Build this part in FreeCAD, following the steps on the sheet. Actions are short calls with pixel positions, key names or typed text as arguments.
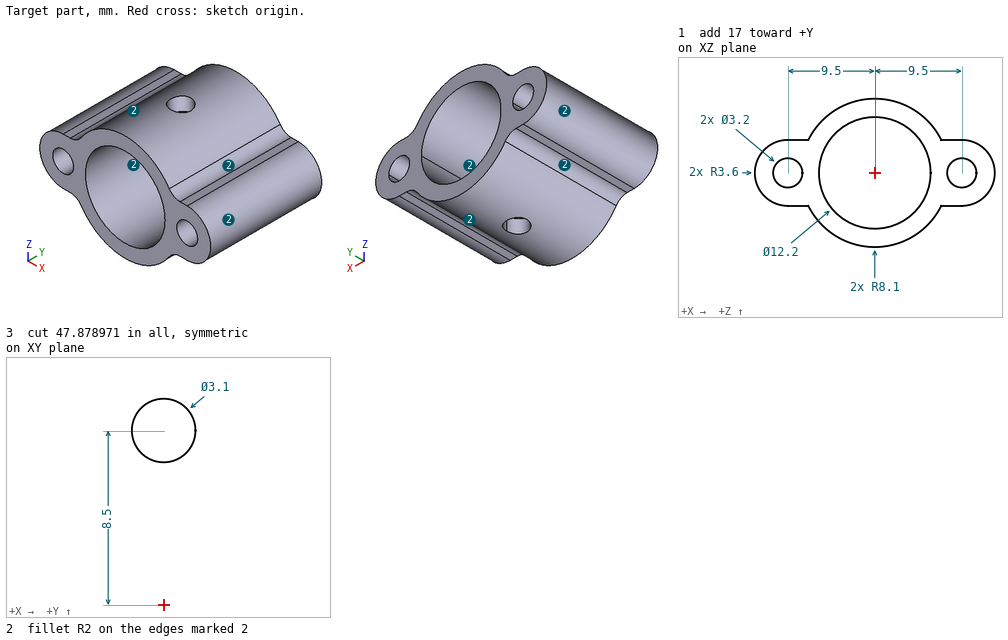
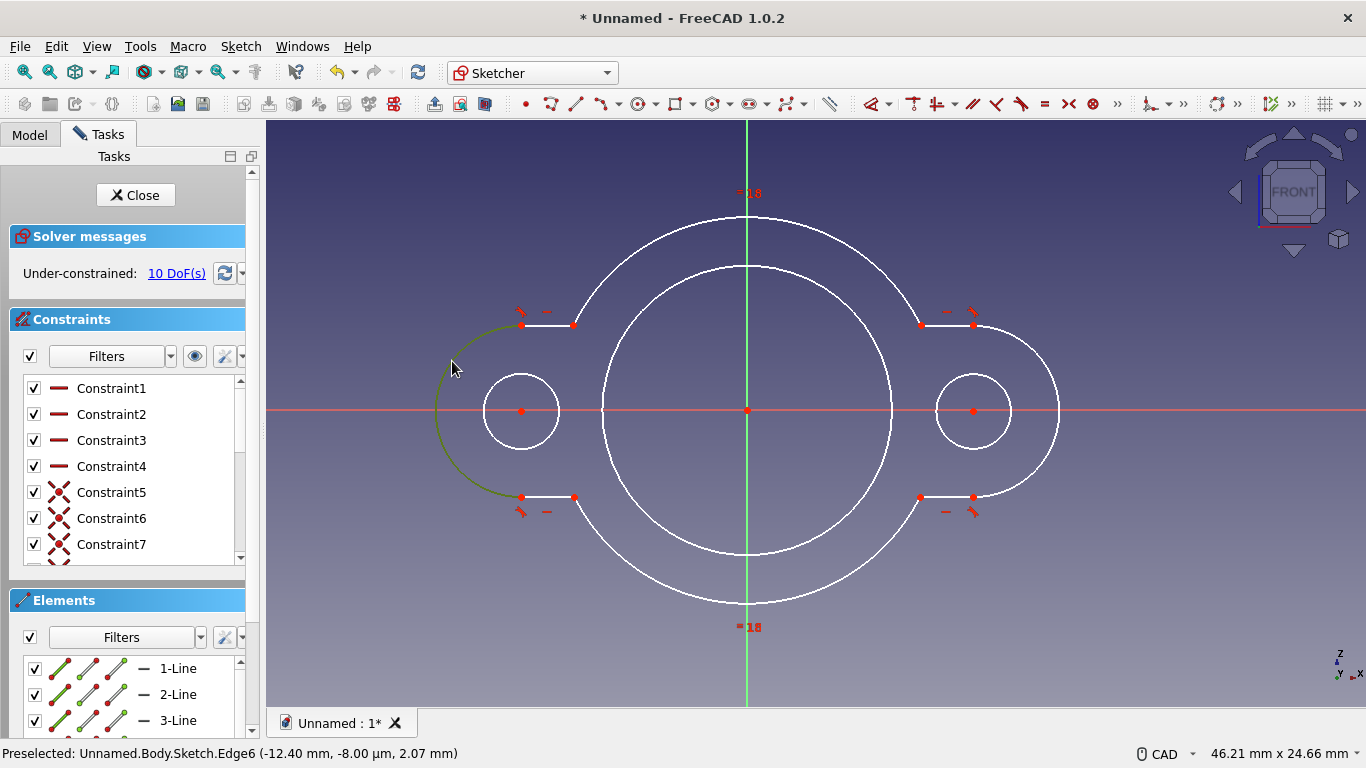
click(1043, 462)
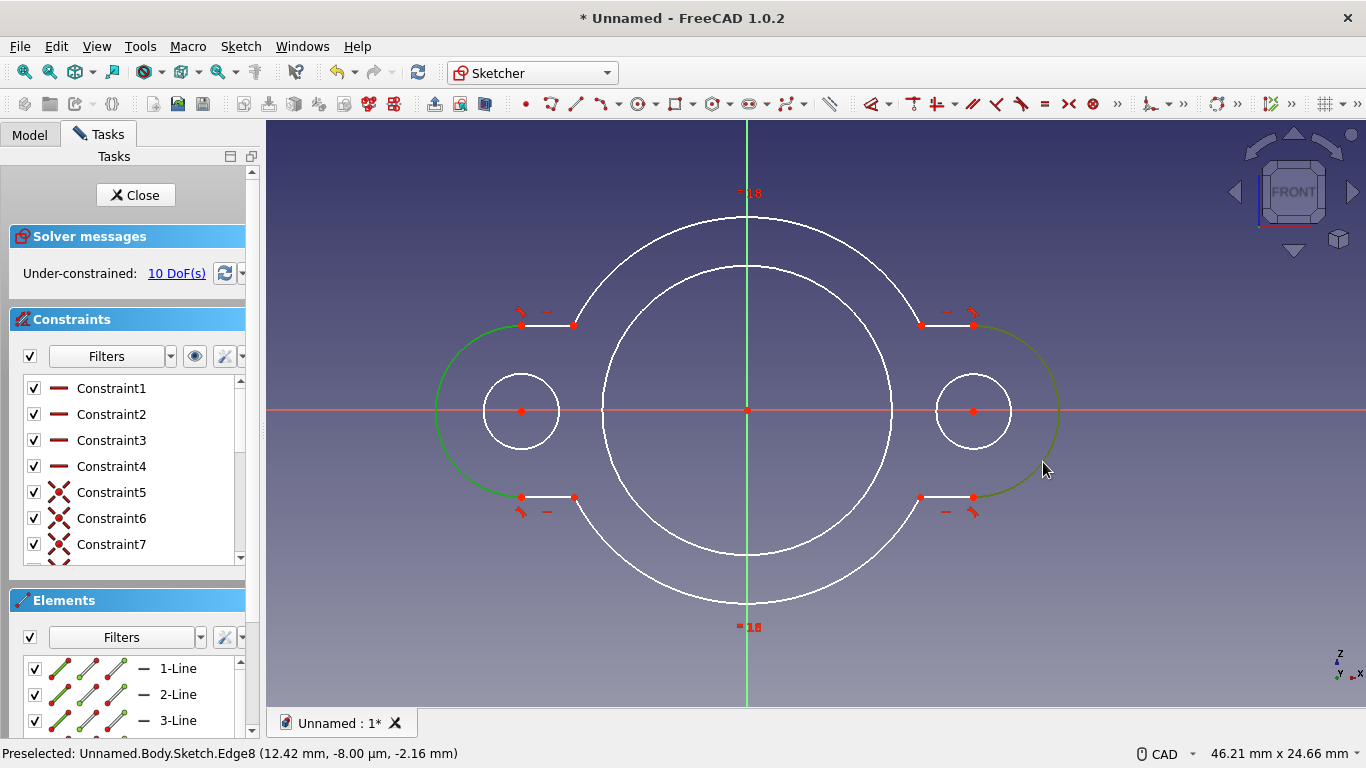
key(e)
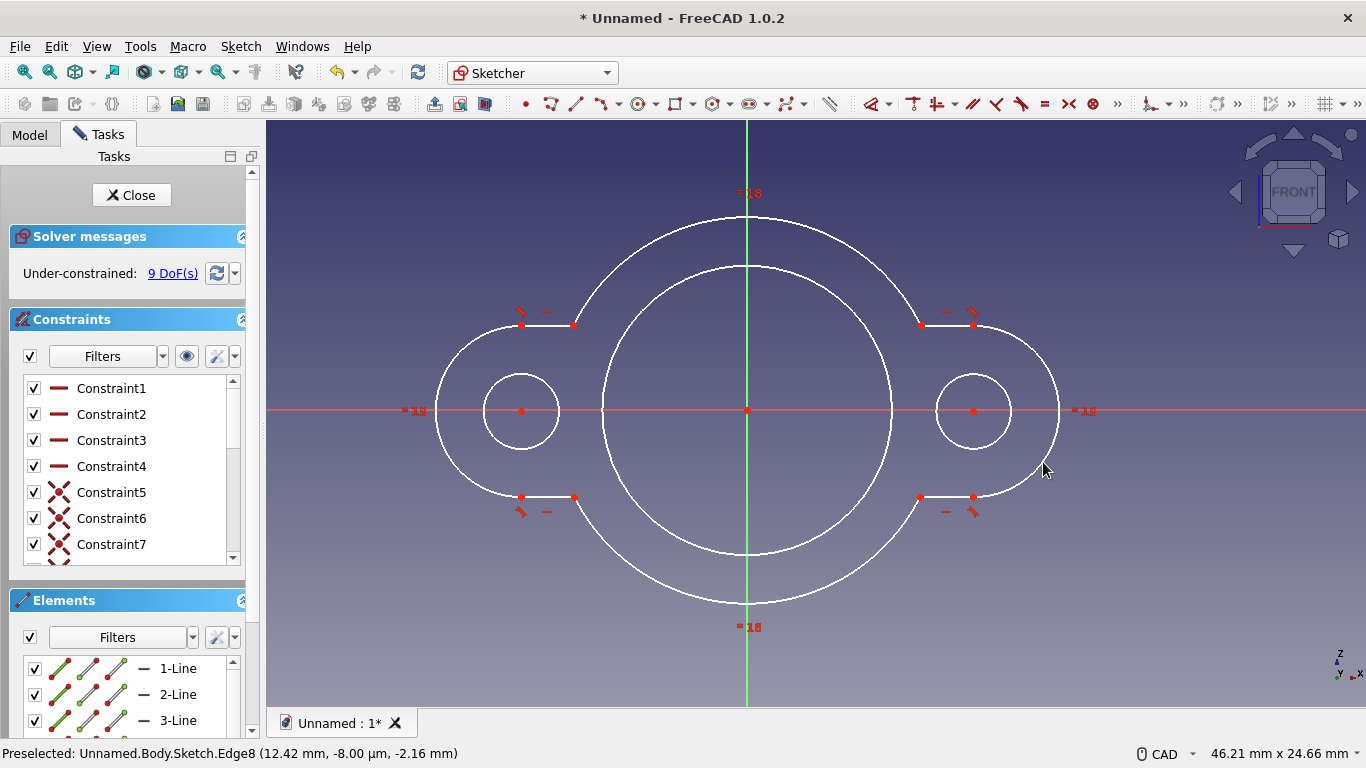
click(548, 385)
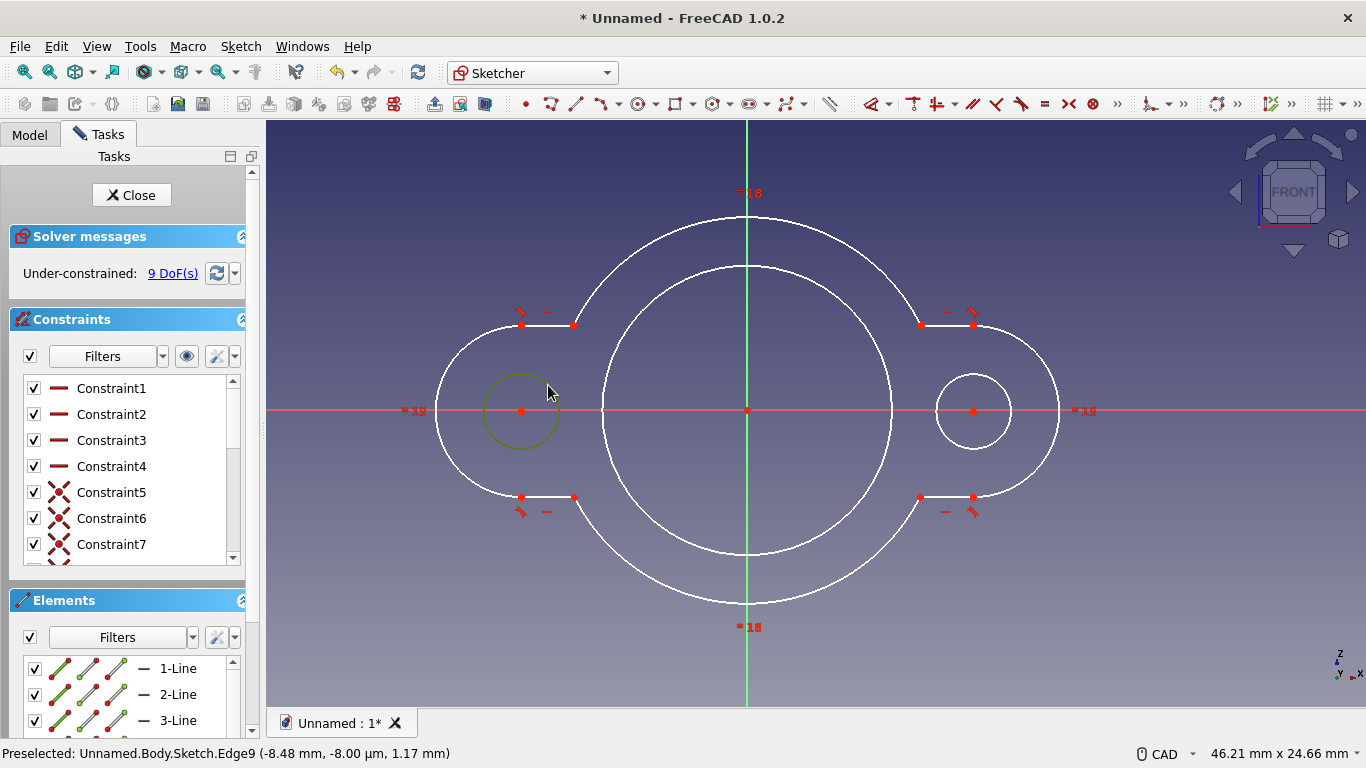
click(1000, 385)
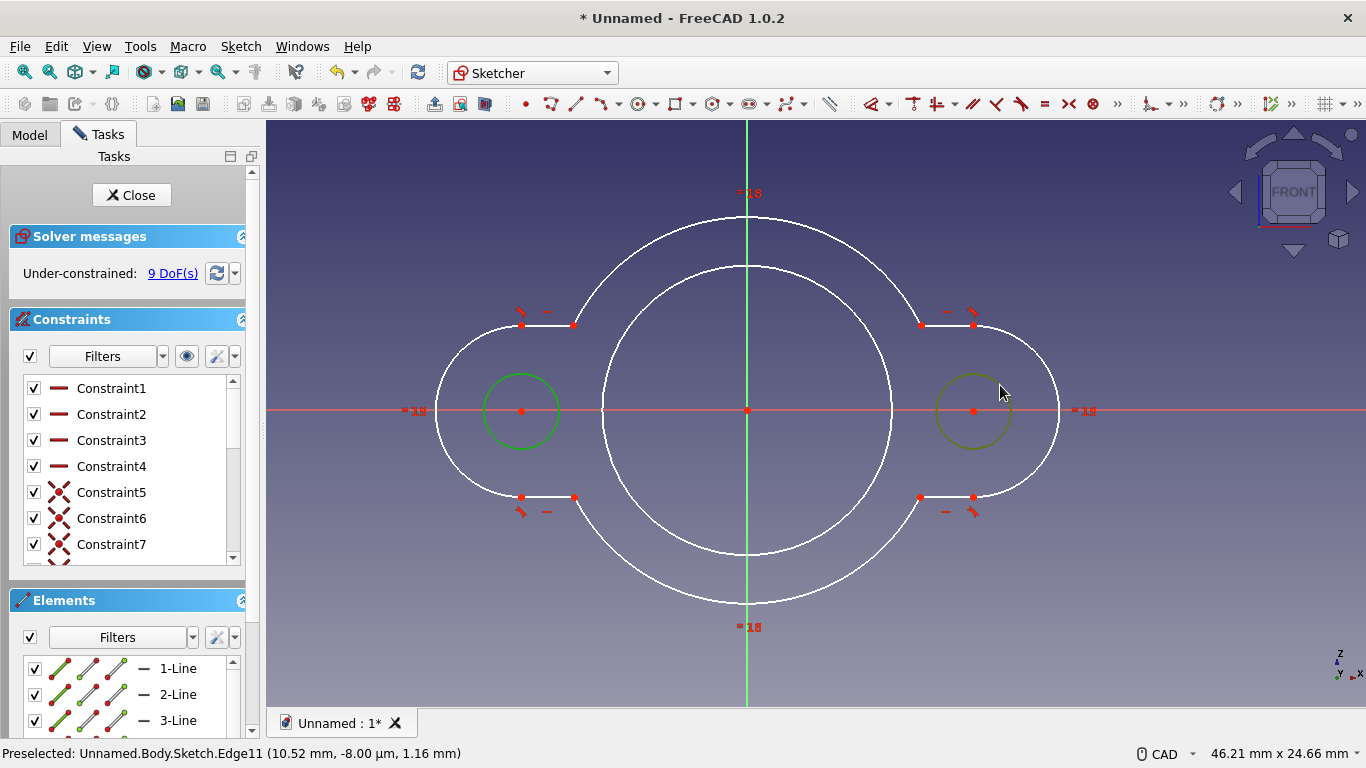
key(e)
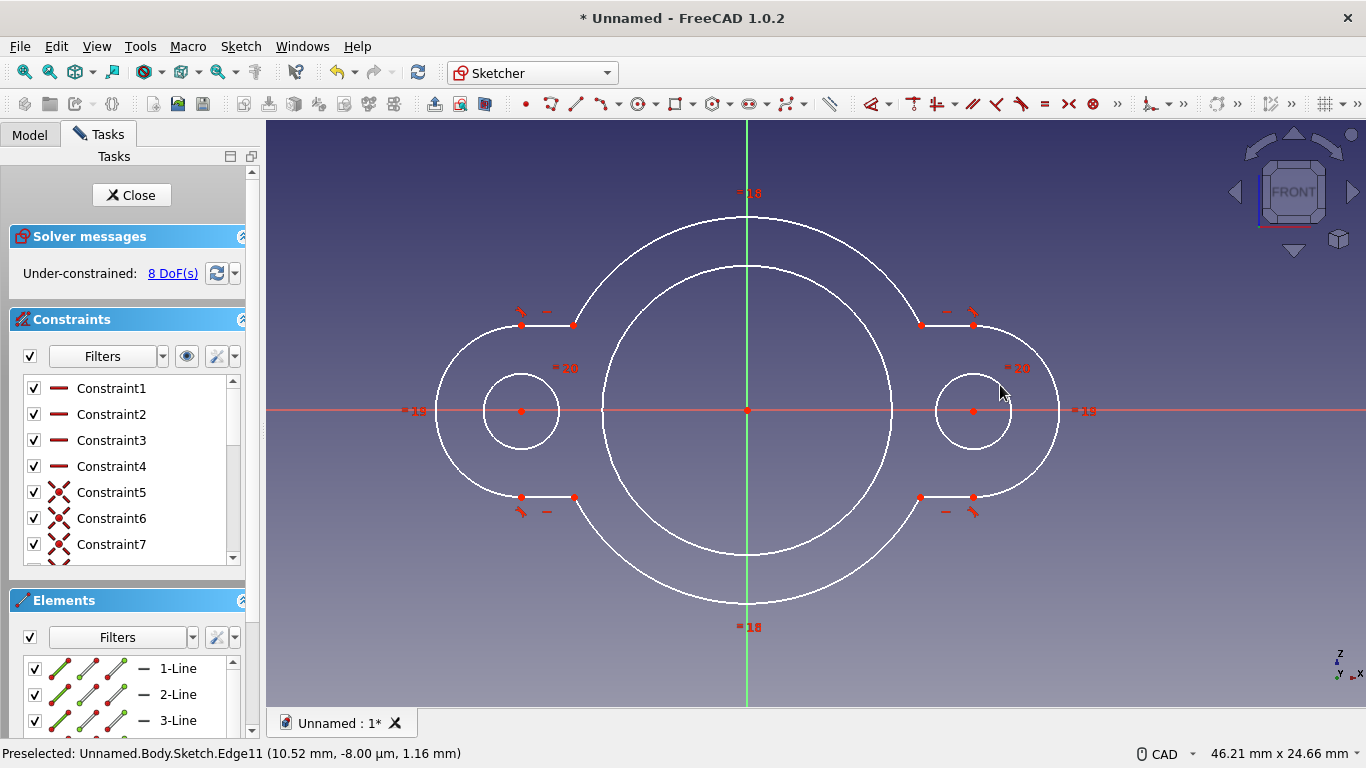
click(521, 412)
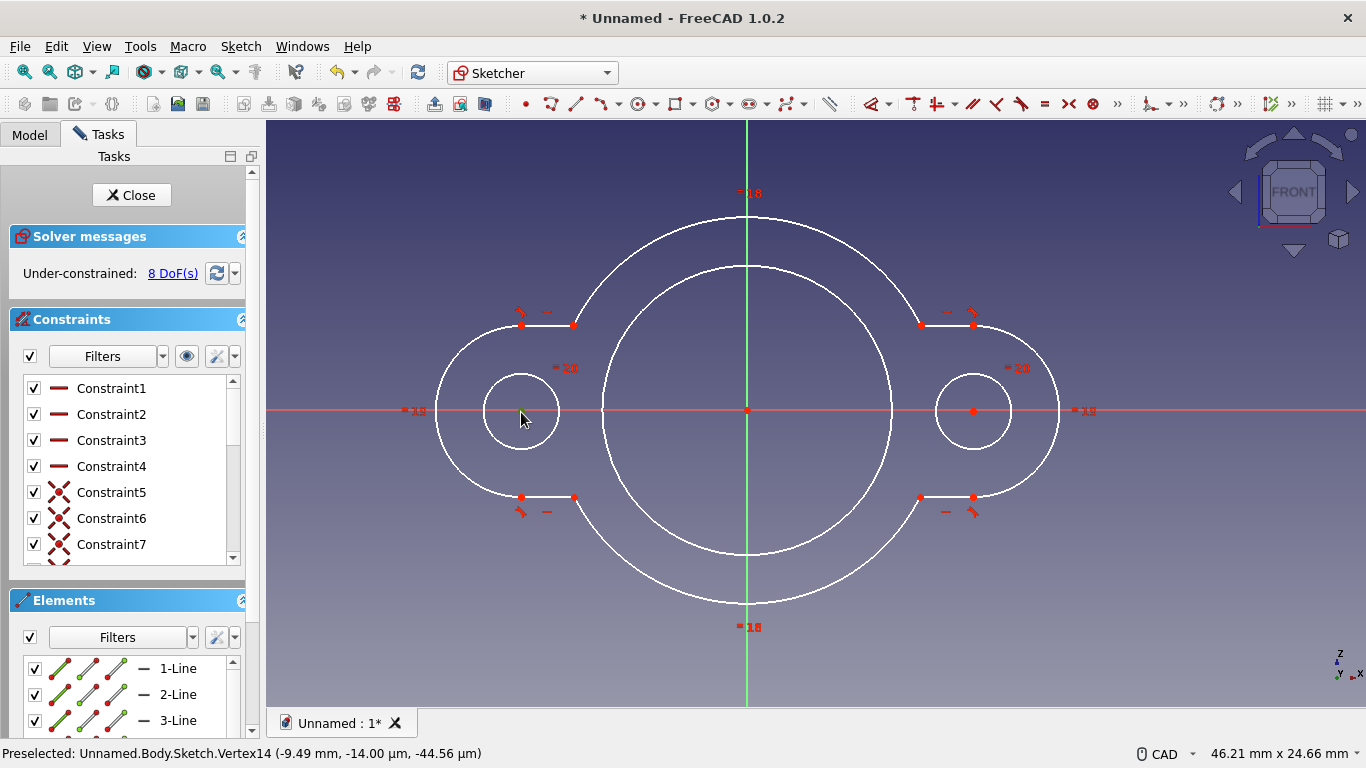
click(359, 410)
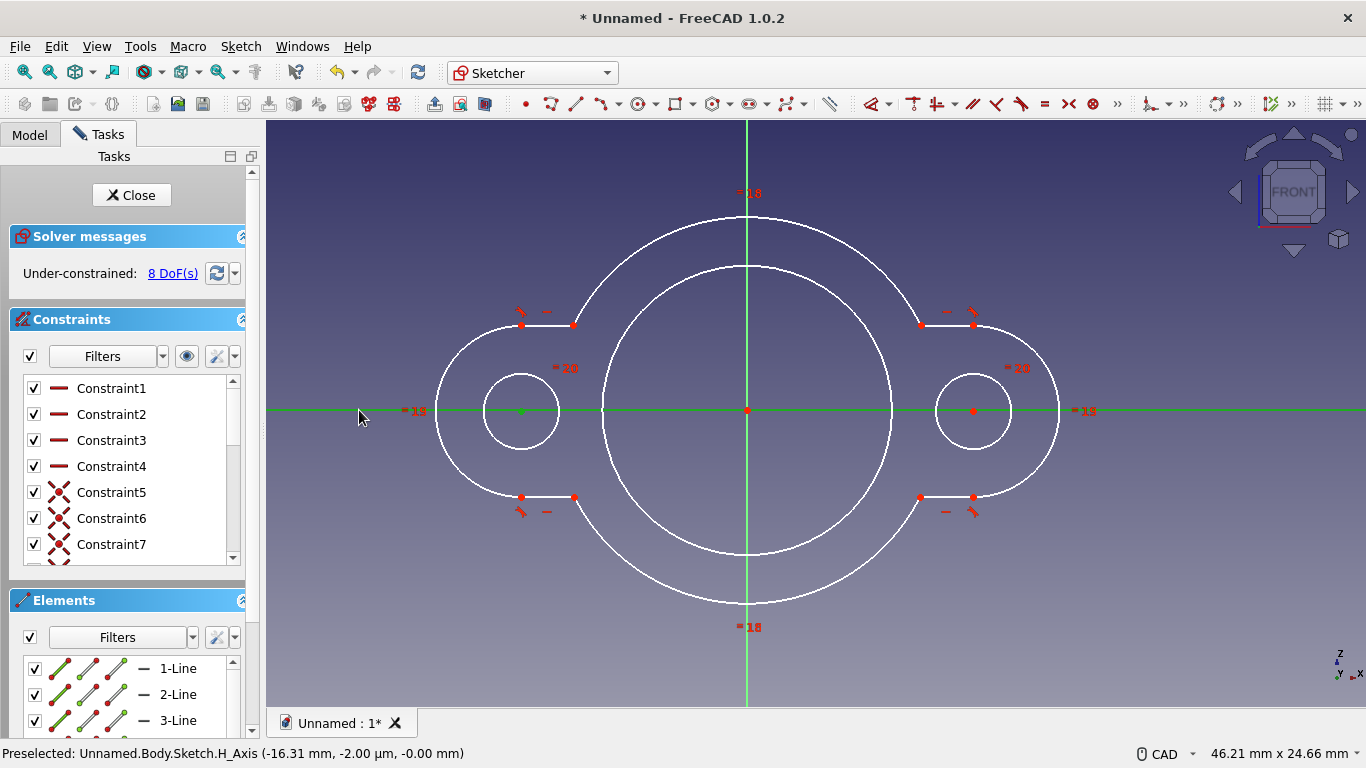
key(c)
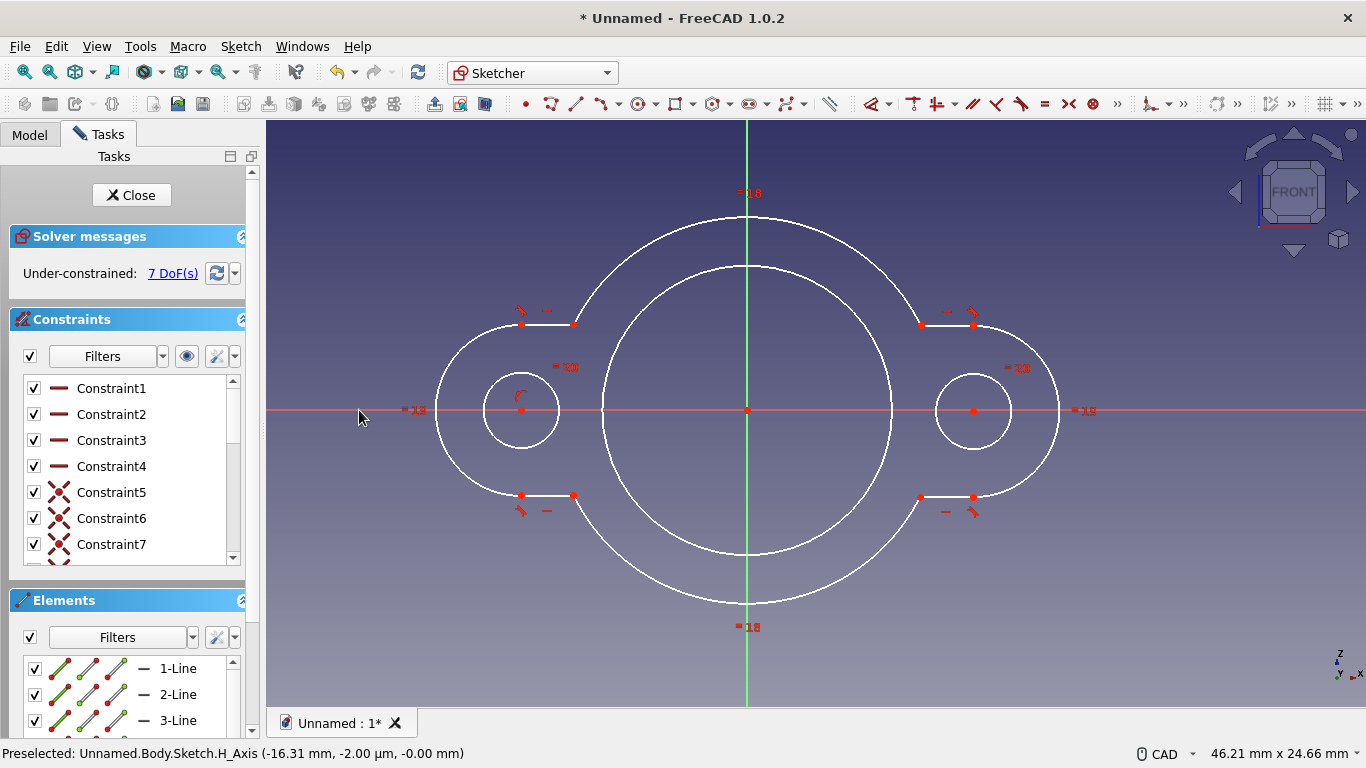
click(974, 412)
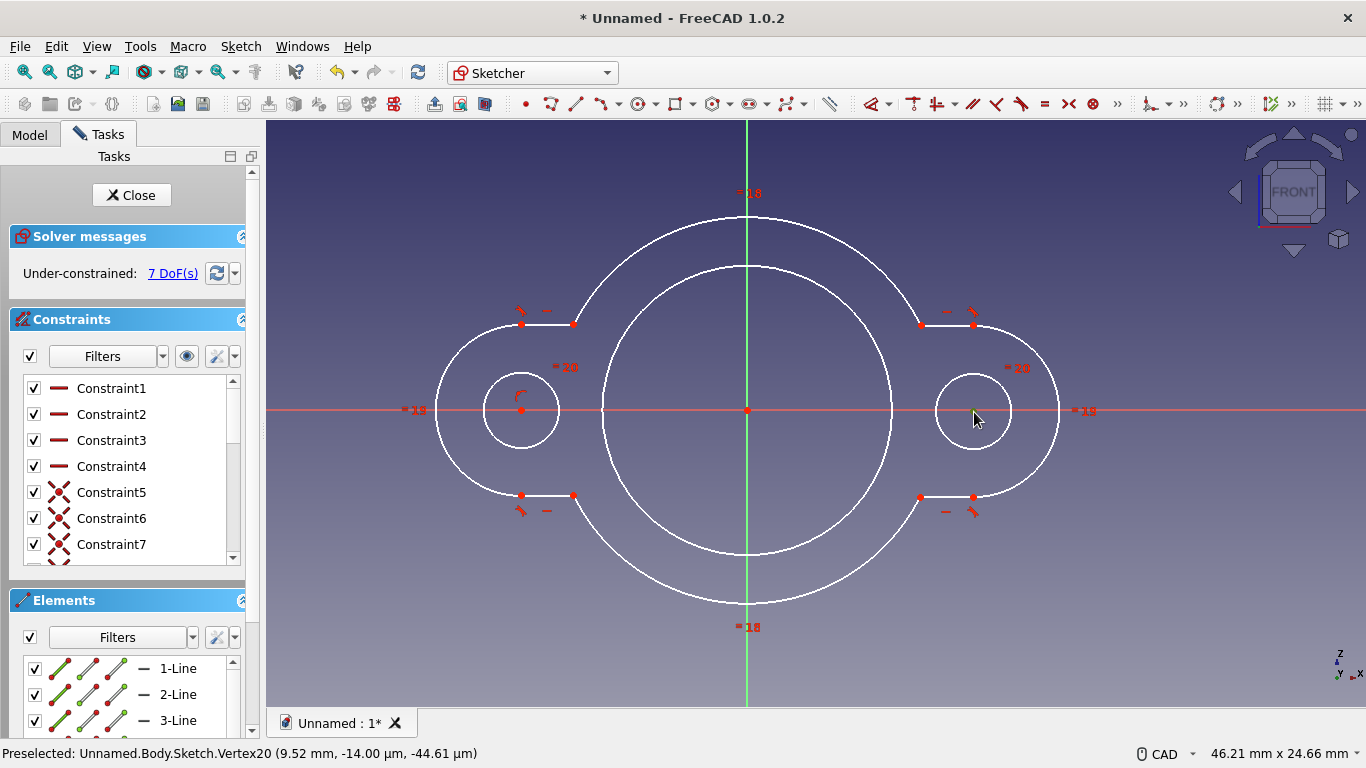
click(359, 410)